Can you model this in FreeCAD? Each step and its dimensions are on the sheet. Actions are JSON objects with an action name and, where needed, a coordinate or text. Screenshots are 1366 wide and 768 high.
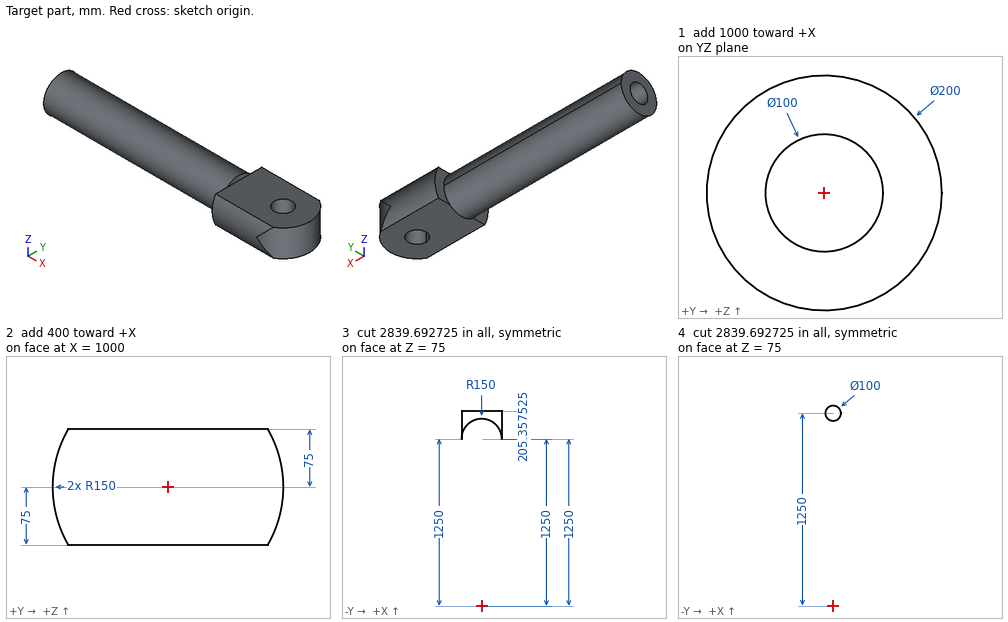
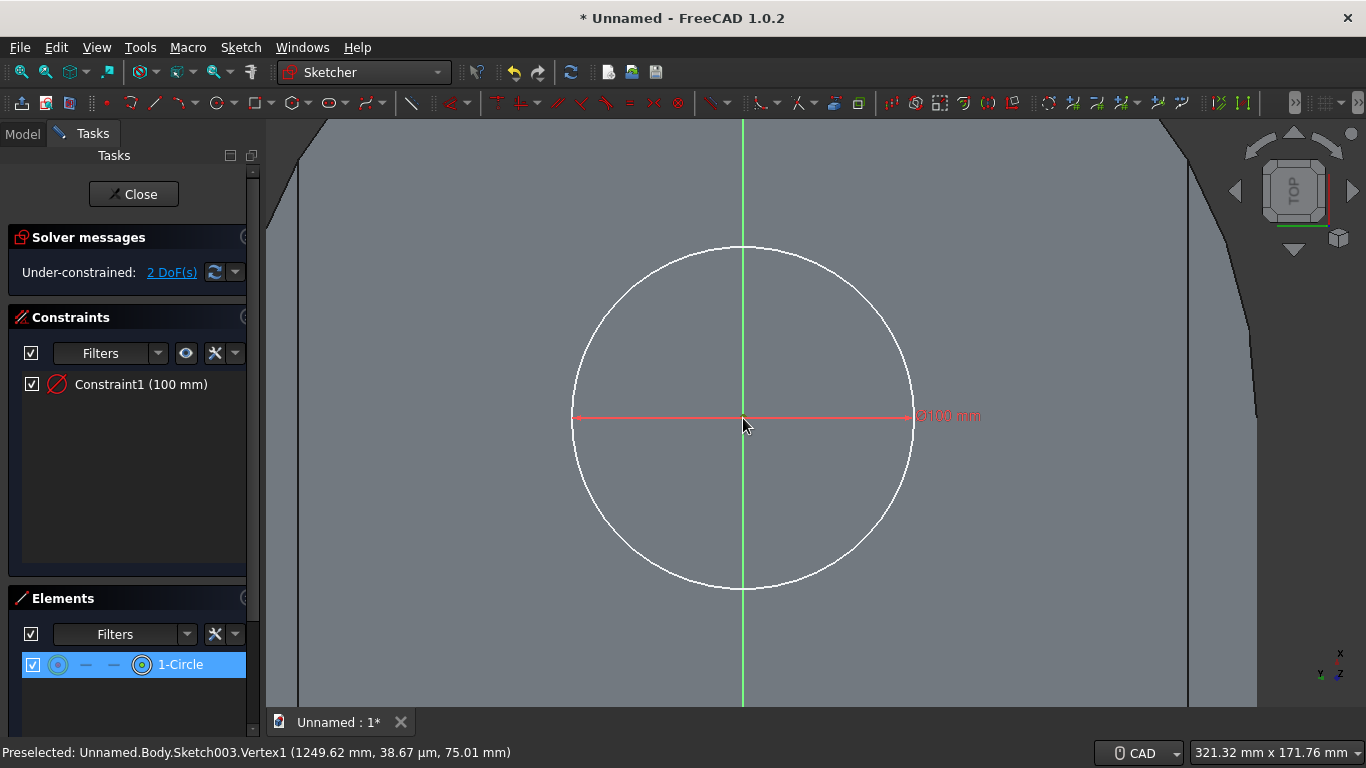
{"action": "left_click", "coordinate": [743, 641]}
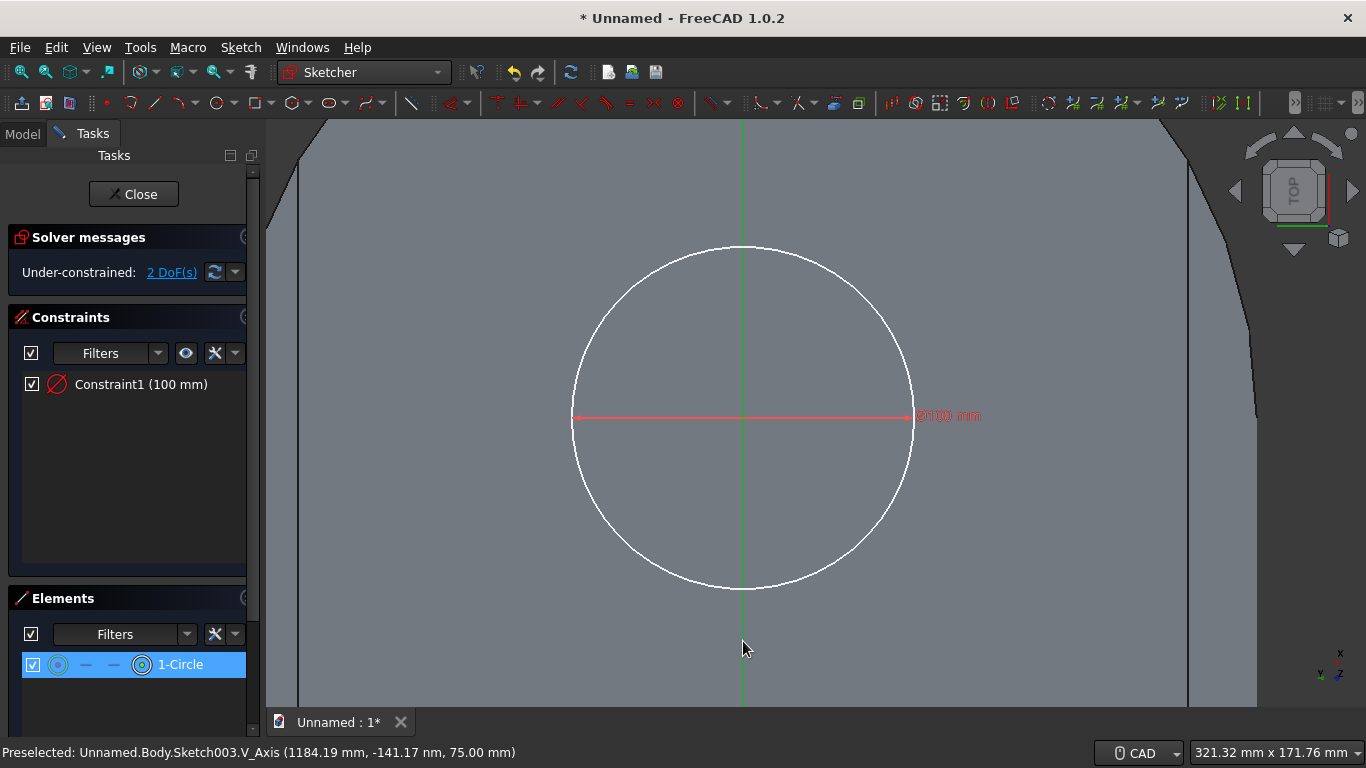
{"action": "left_click", "coordinate": [498, 104]}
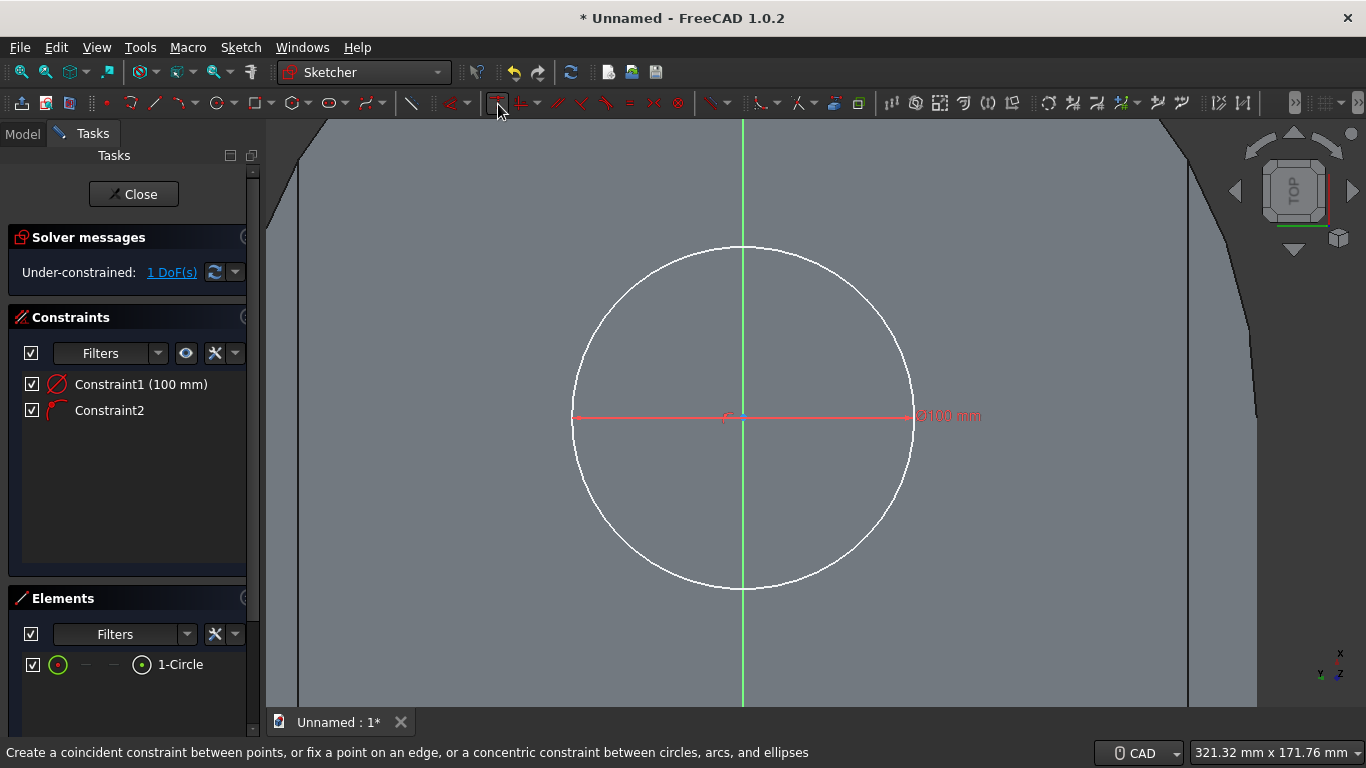
{"action": "left_click", "coordinate": [450, 104]}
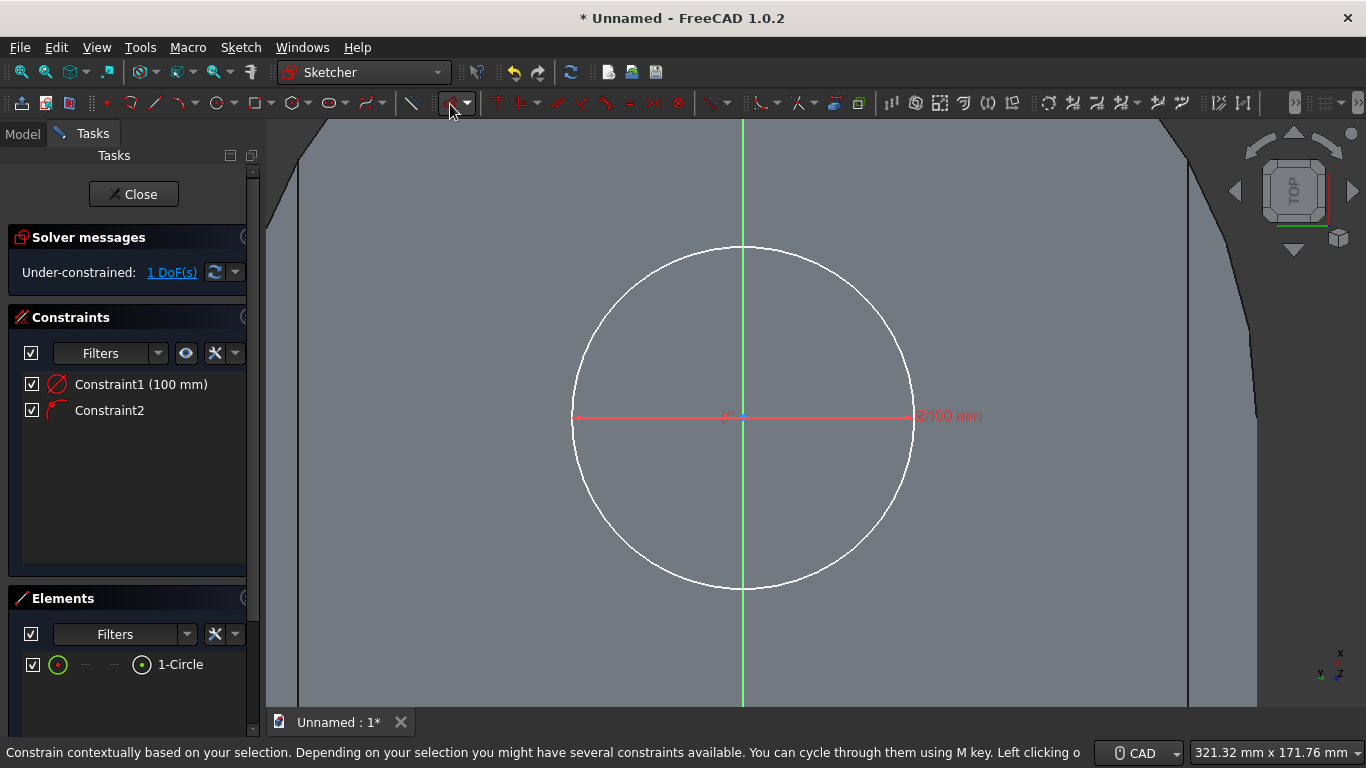
{"action": "left_click", "coordinate": [743, 418]}
{"action": "left_click", "coordinate": [777, 549]}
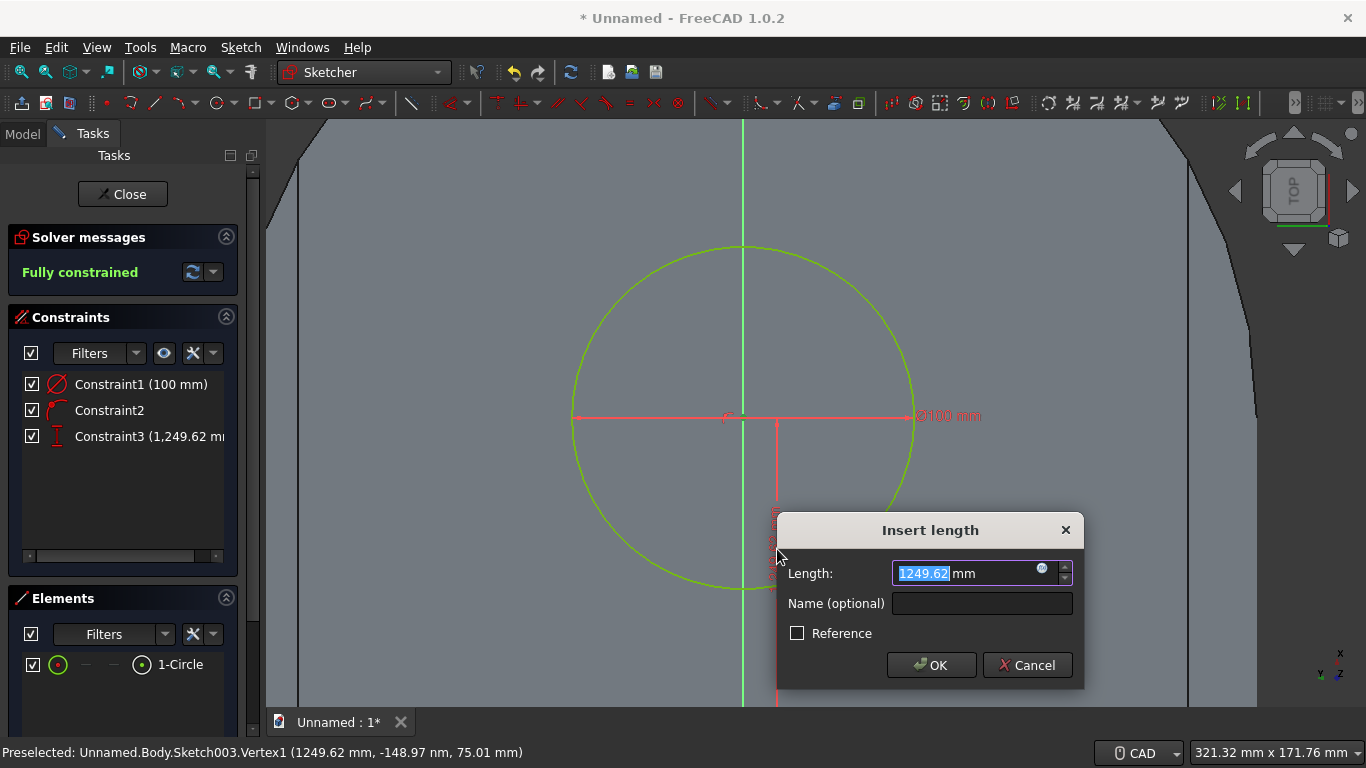
{"action": "type", "text": "1250"}
{"action": "key", "text": "Return"}
{"action": "key", "text": "Escape"}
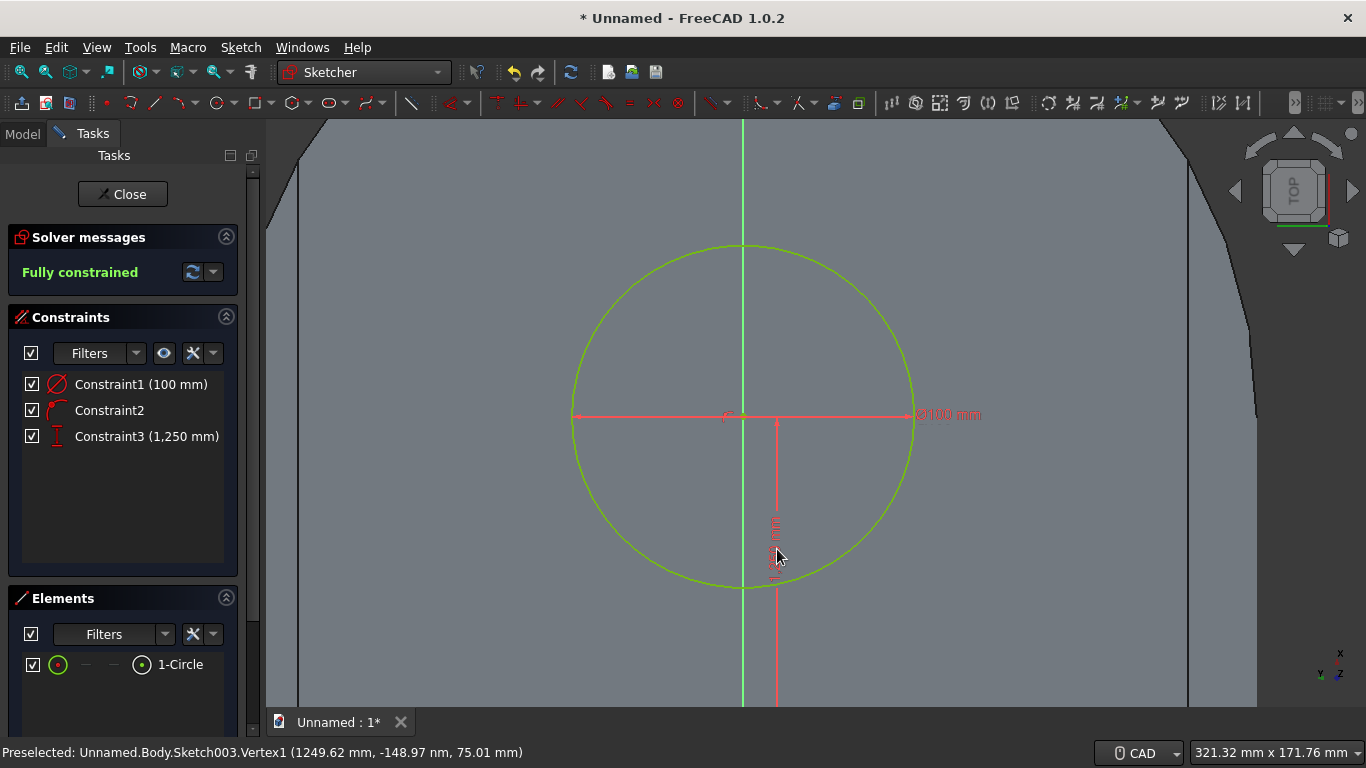
{"action": "left_click", "coordinate": [123, 194]}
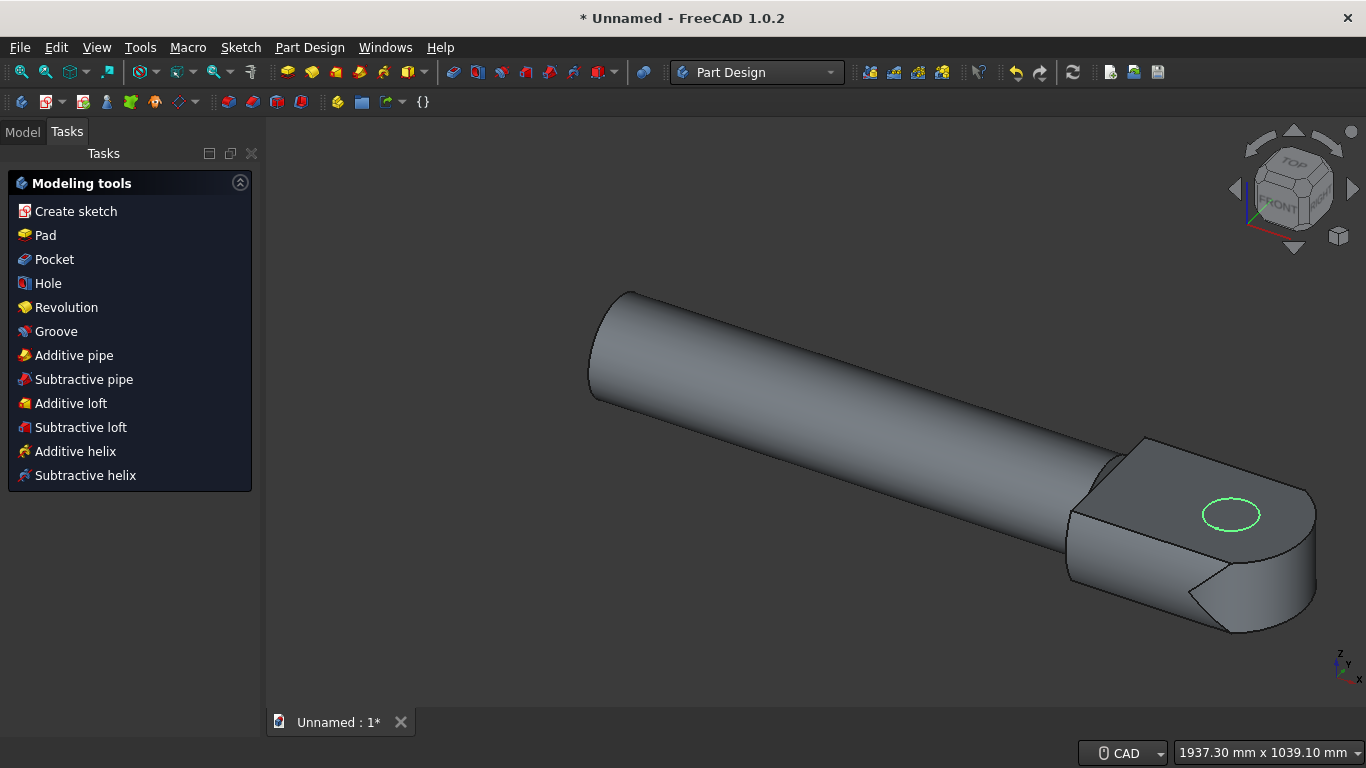
{"action": "left_click", "coordinate": [454, 72]}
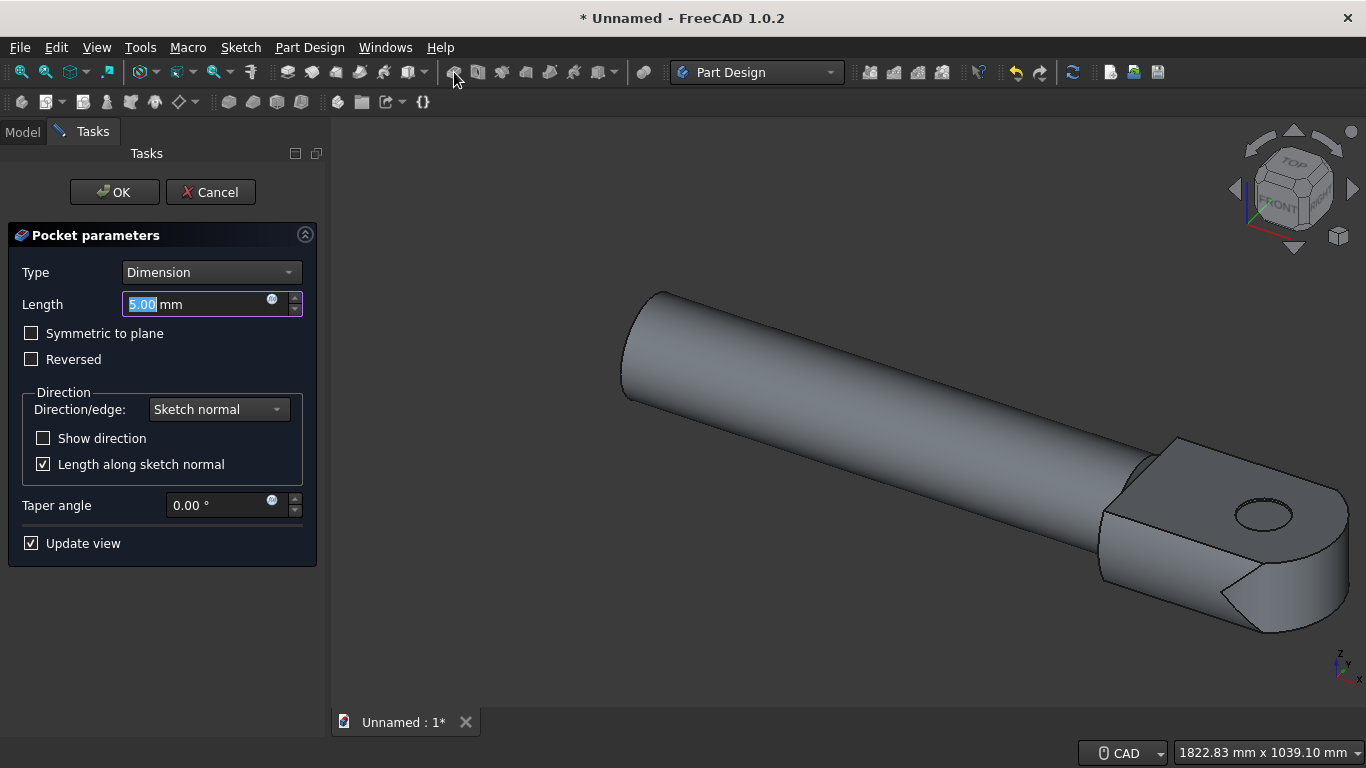
{"action": "type", "text": "2839.692725"}
{"action": "key", "text": "Tab"}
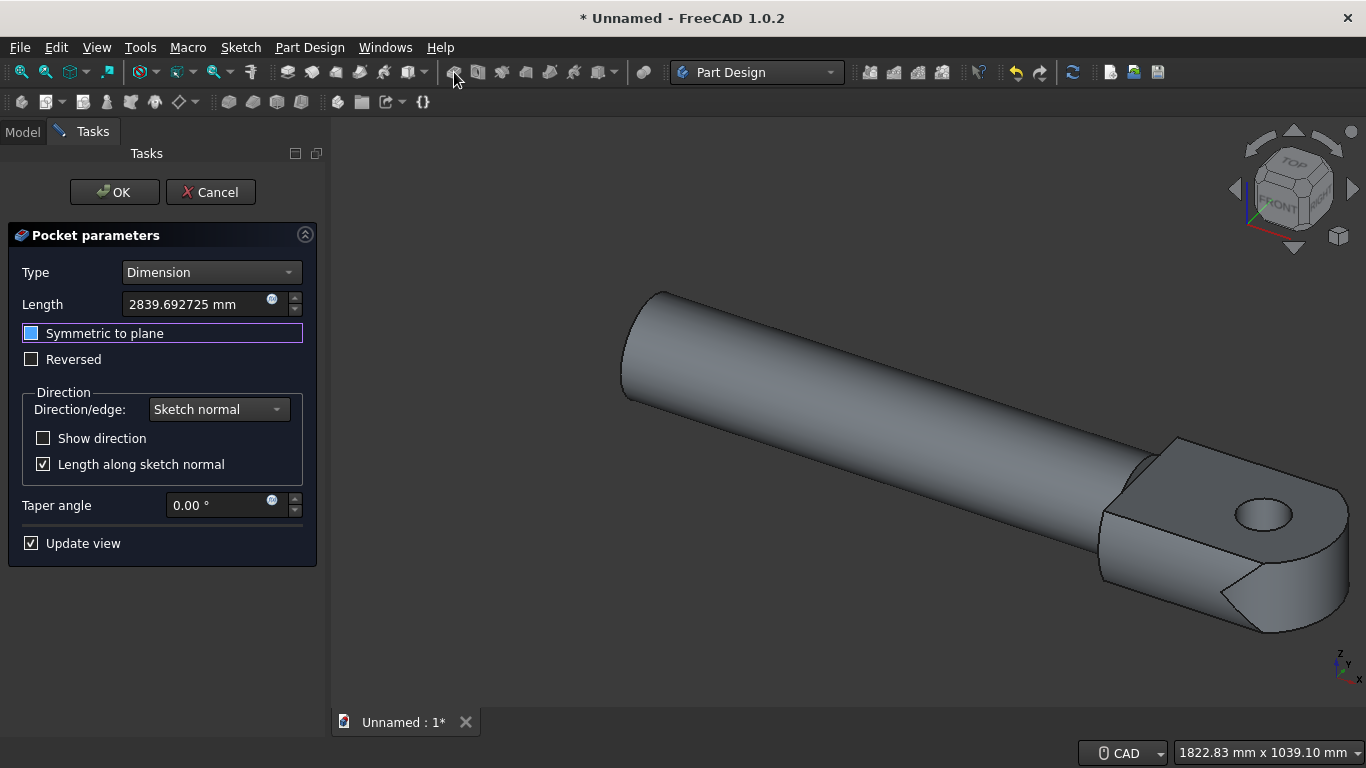
{"action": "left_click", "coordinate": [30, 333]}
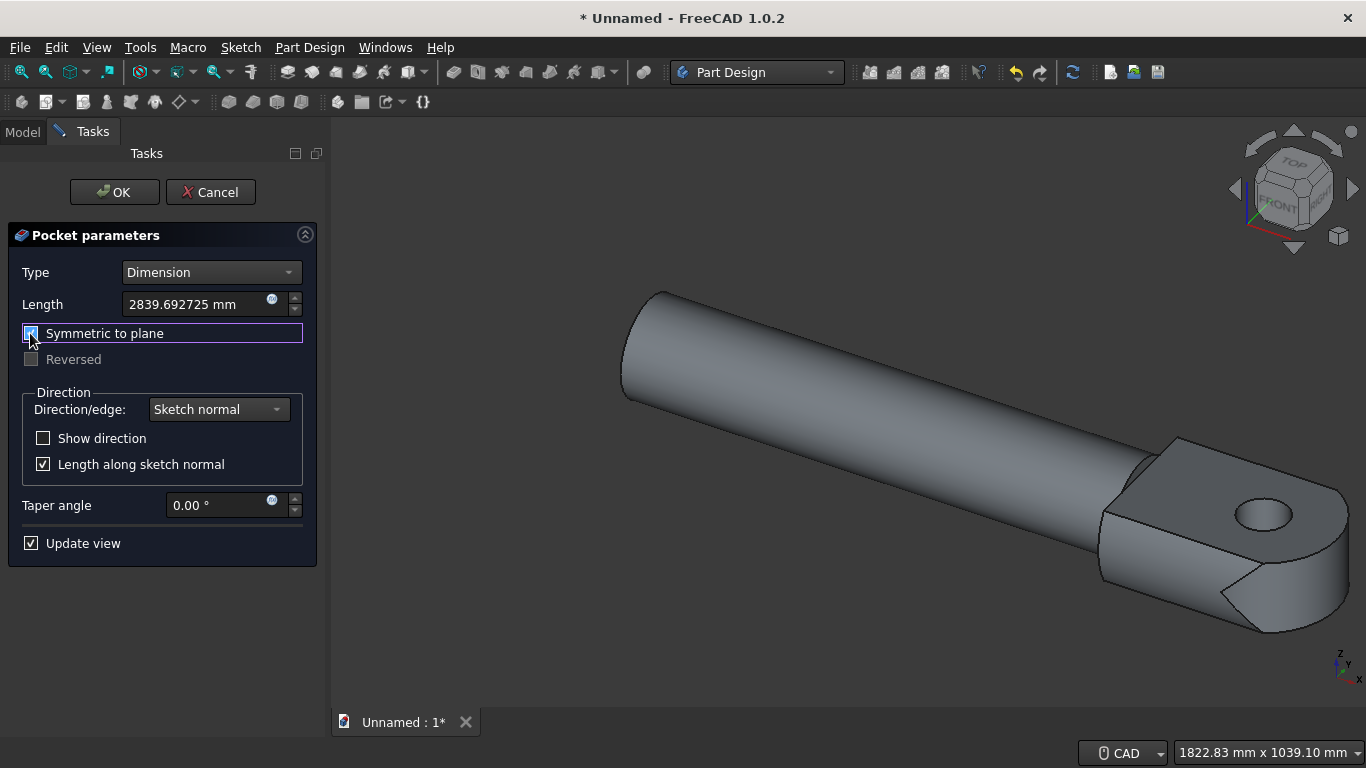
{"action": "left_click", "coordinate": [115, 192]}